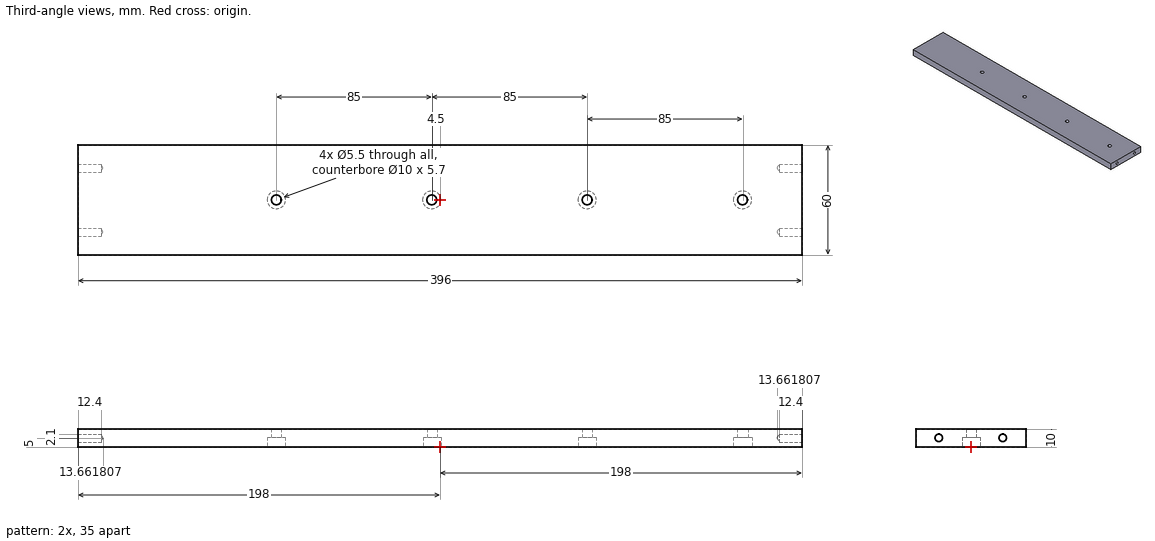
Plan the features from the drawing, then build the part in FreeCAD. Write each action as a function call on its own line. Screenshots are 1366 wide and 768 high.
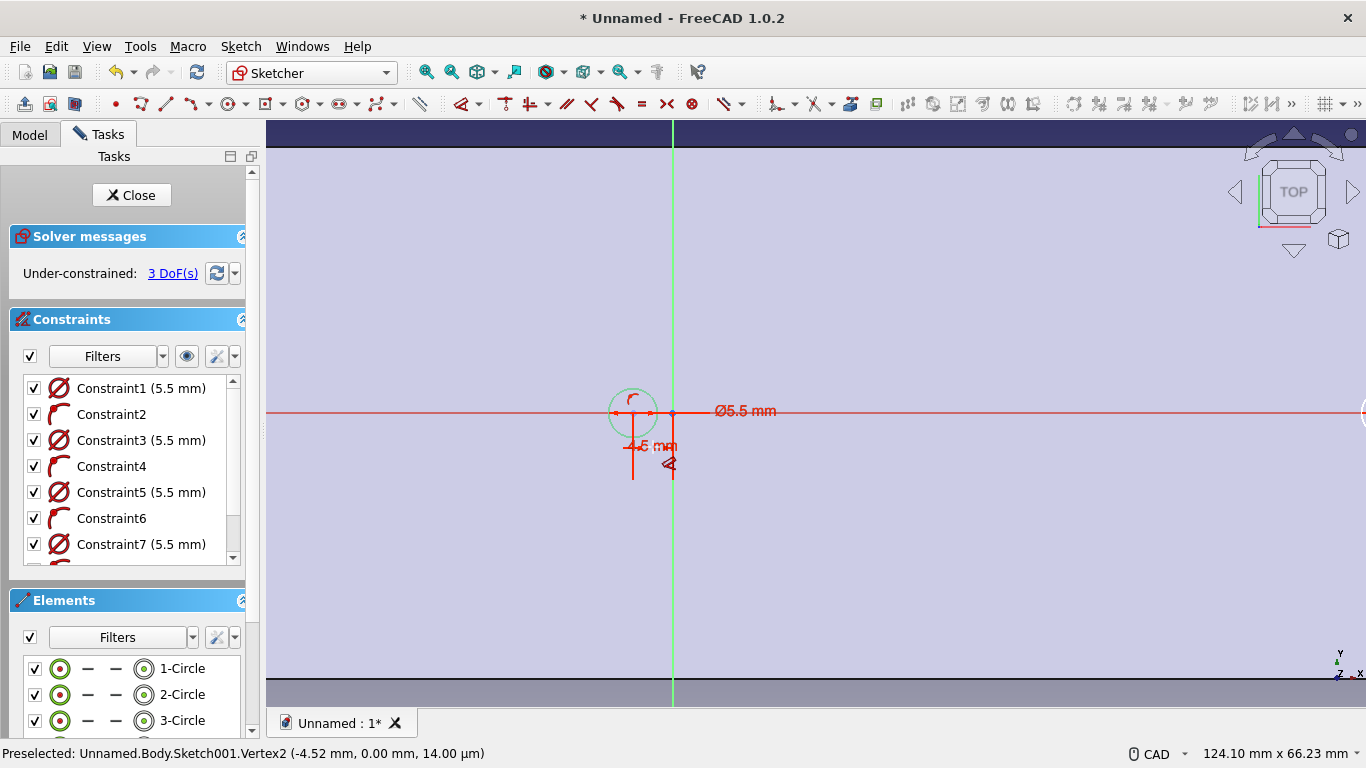
scroll(634, 414, down, 6)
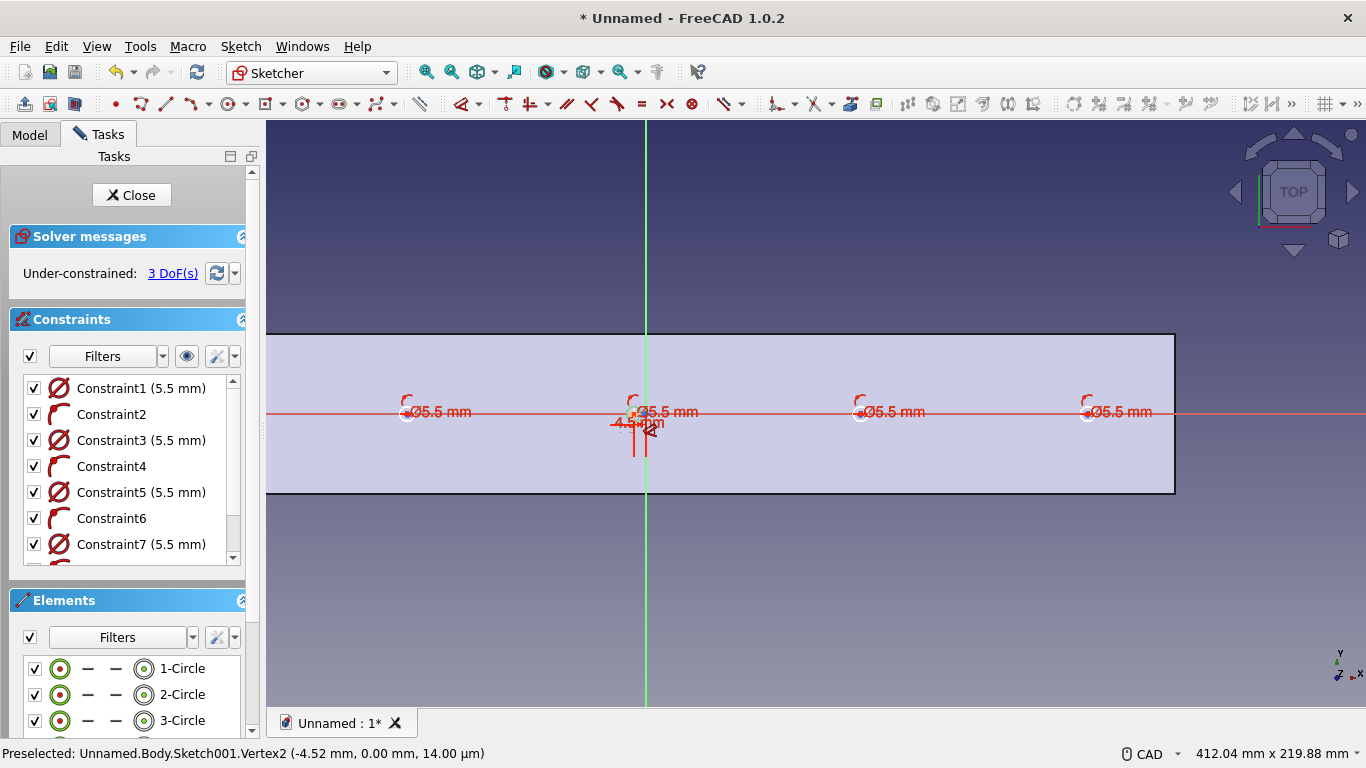
click(407, 414)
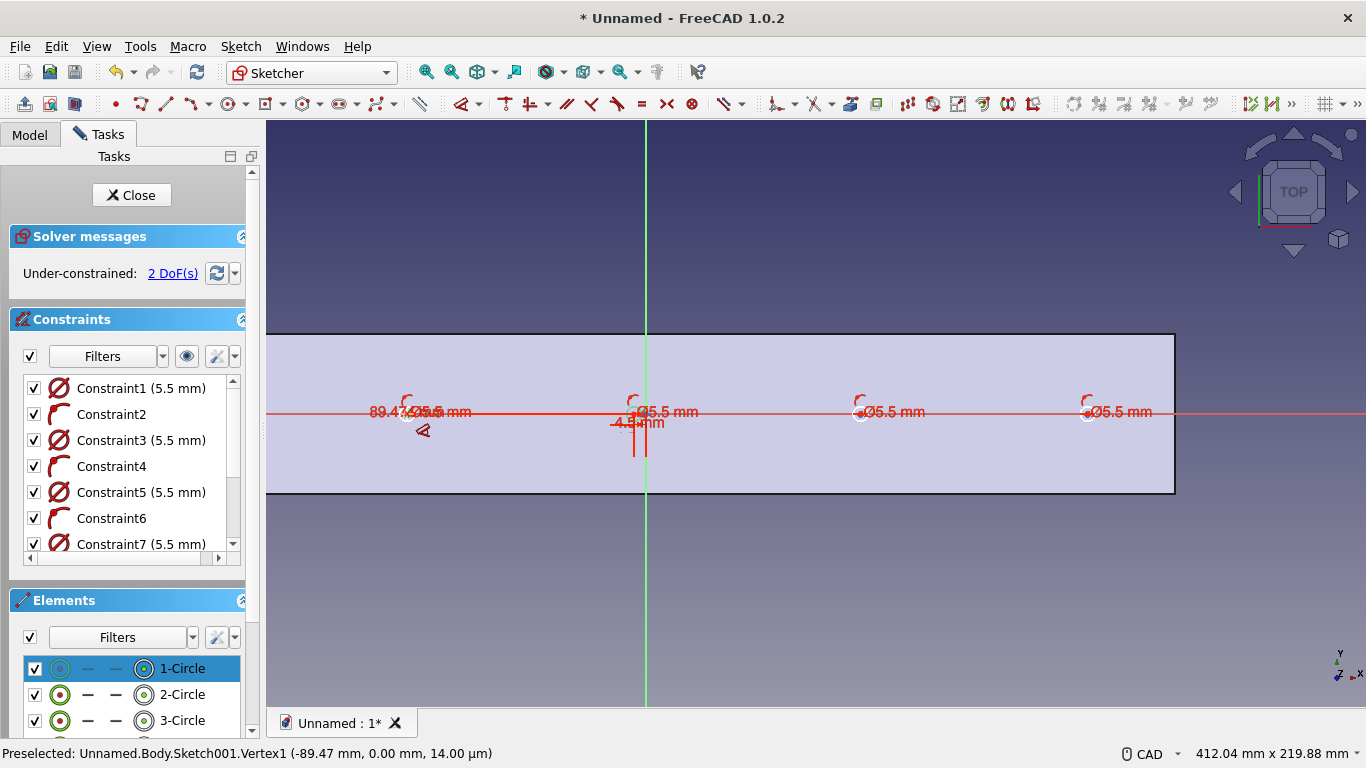
click(634, 414)
click(521, 448)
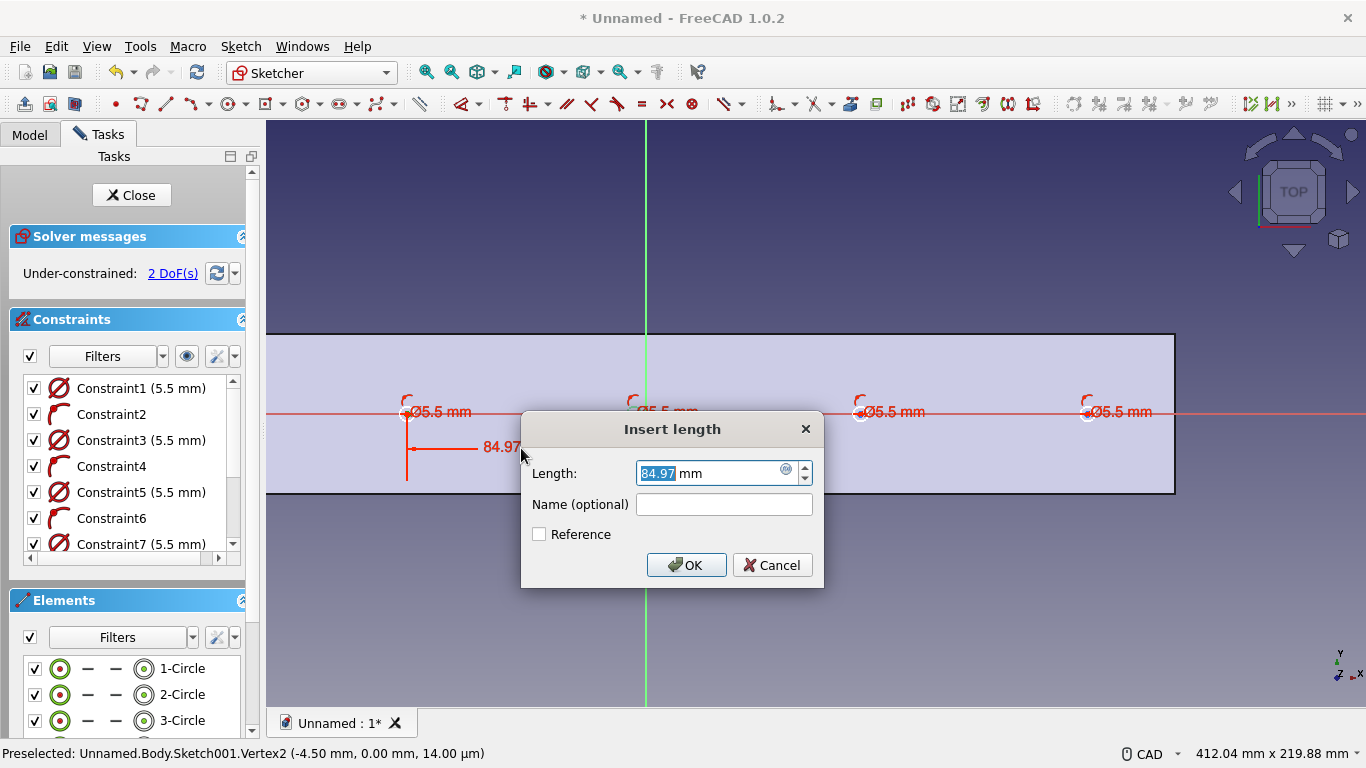
text(85)
key(Return)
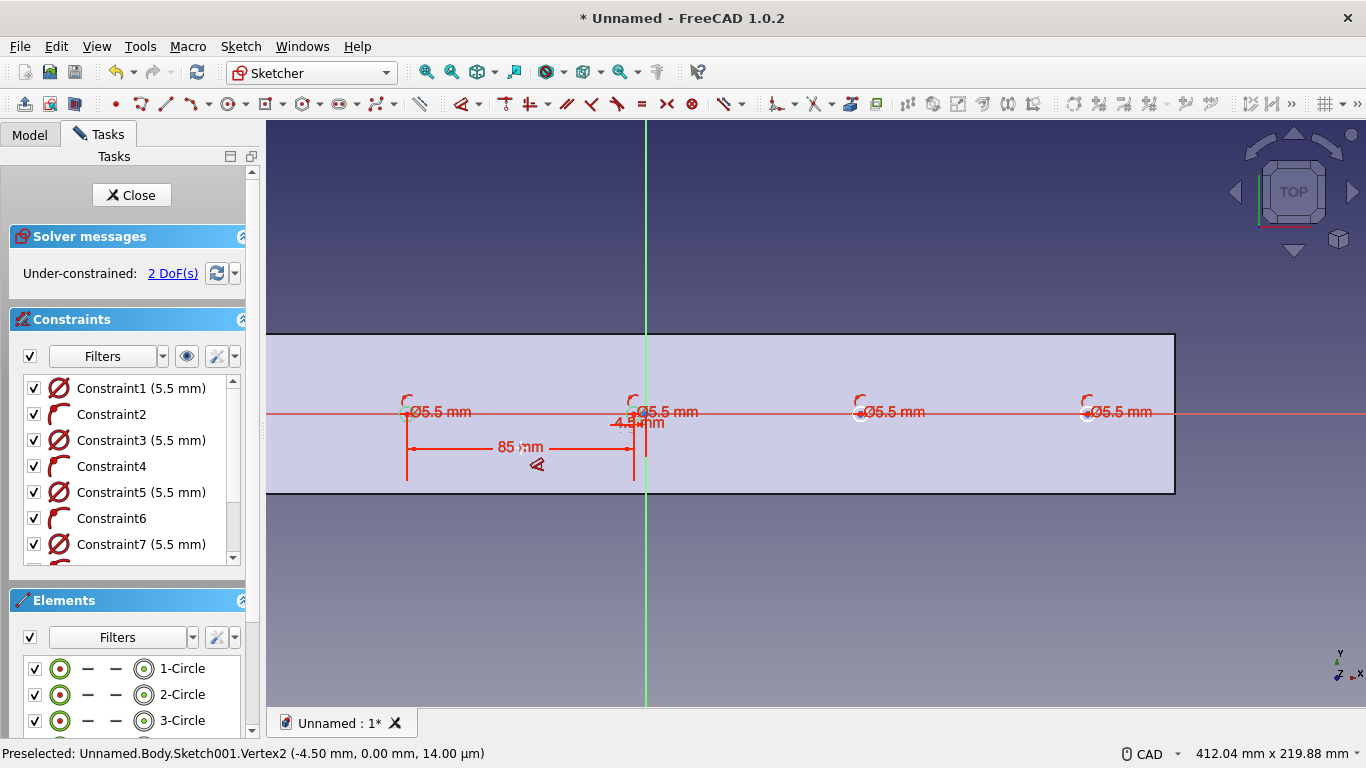
click(634, 414)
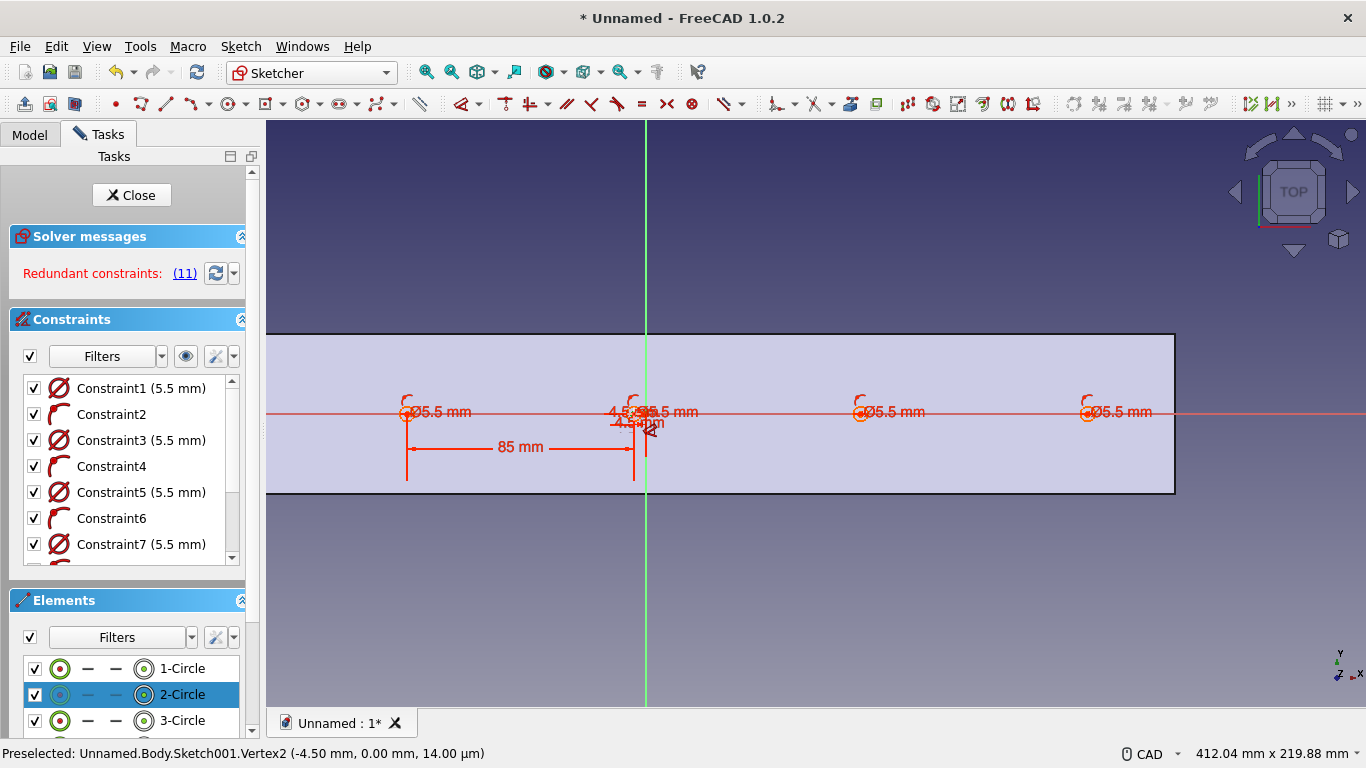
click(861, 414)
click(747, 448)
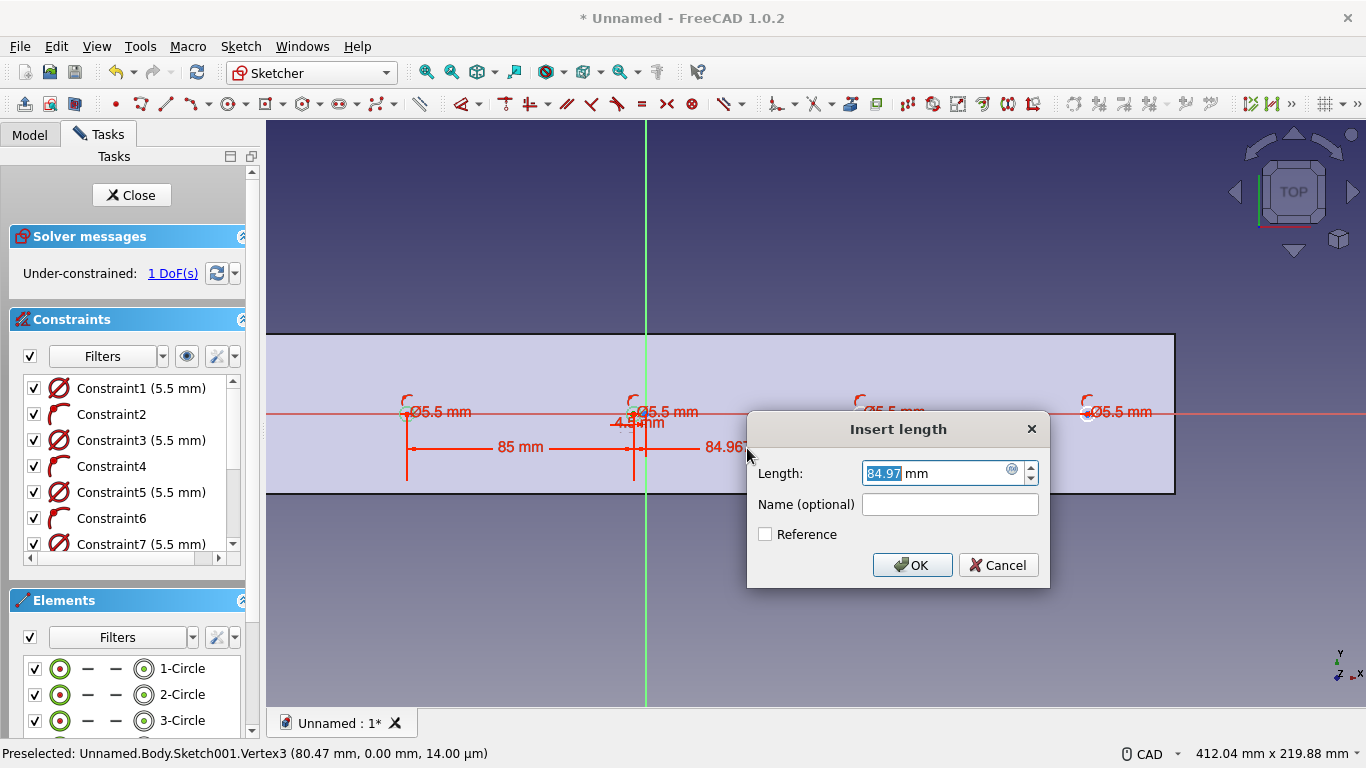
text(85)
key(Return)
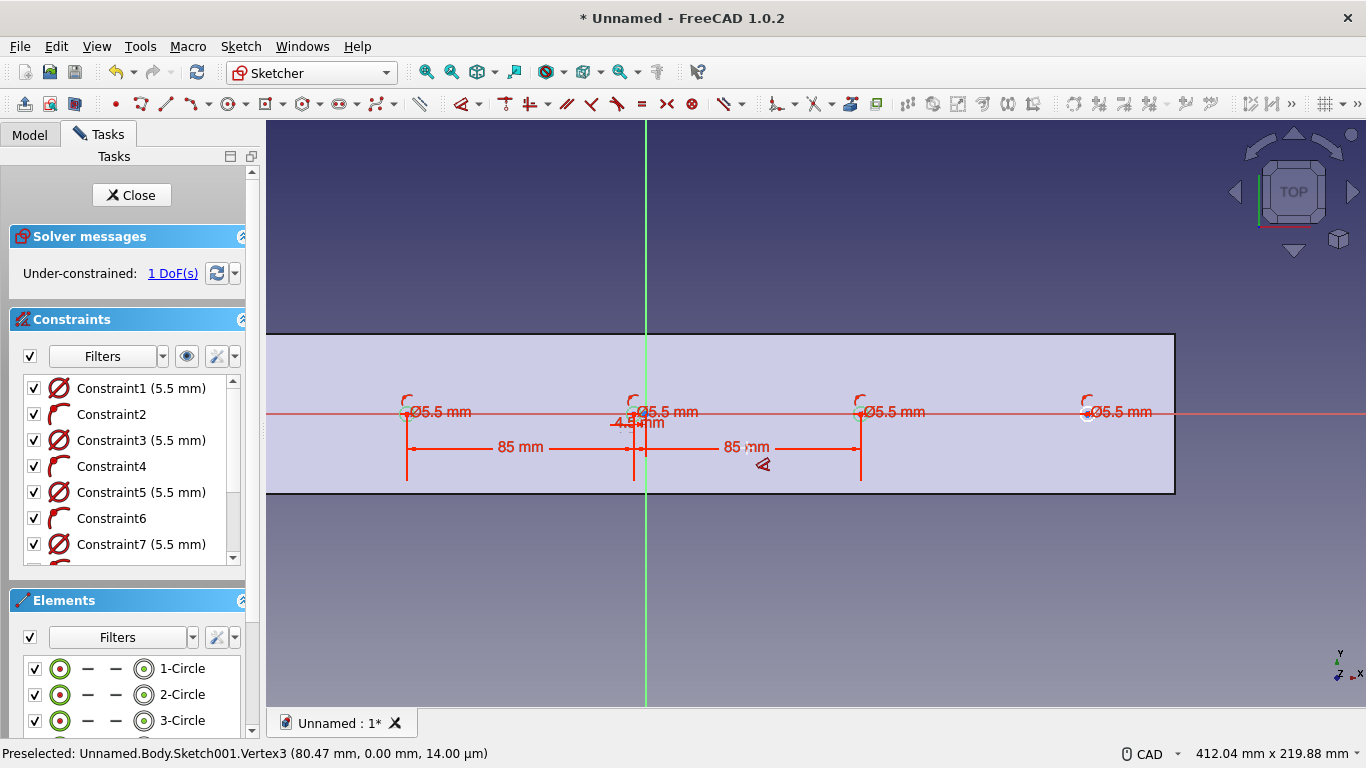
click(861, 414)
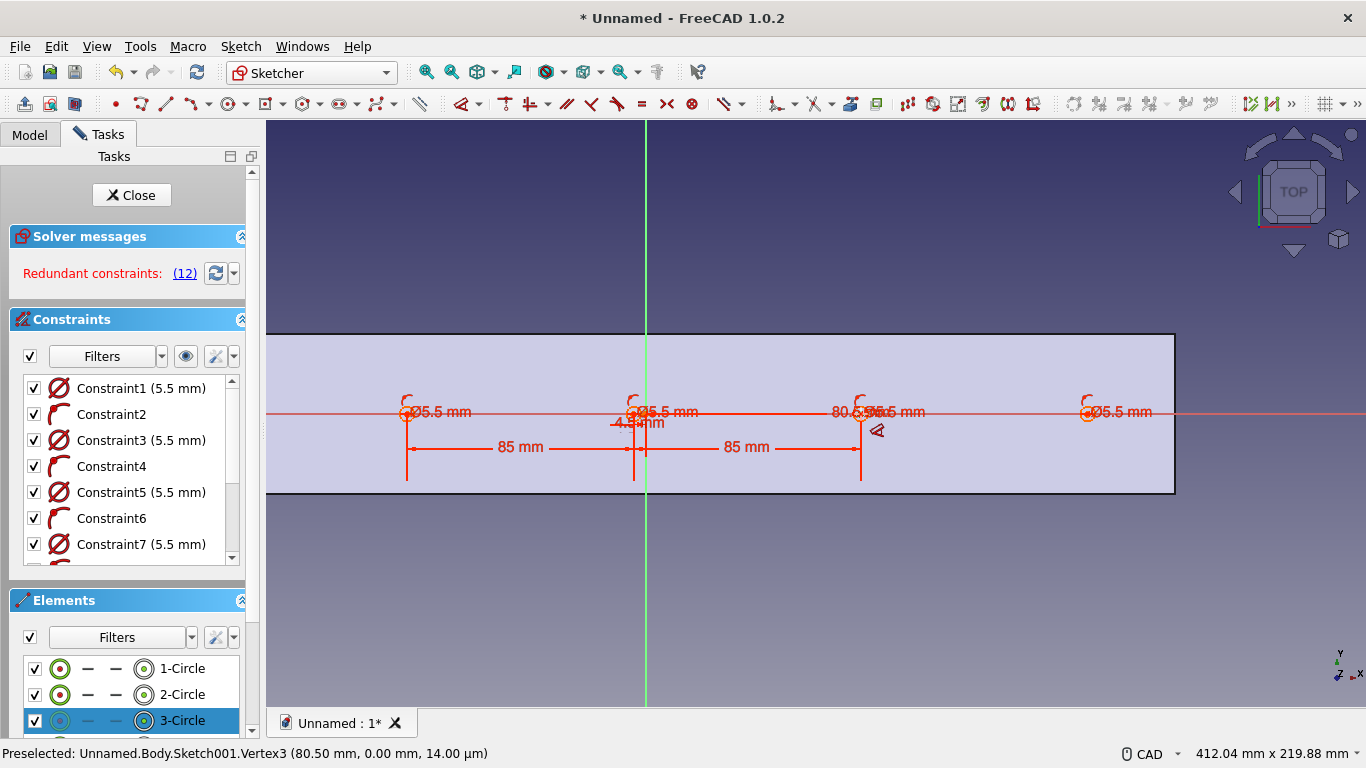
click(1088, 414)
click(974, 448)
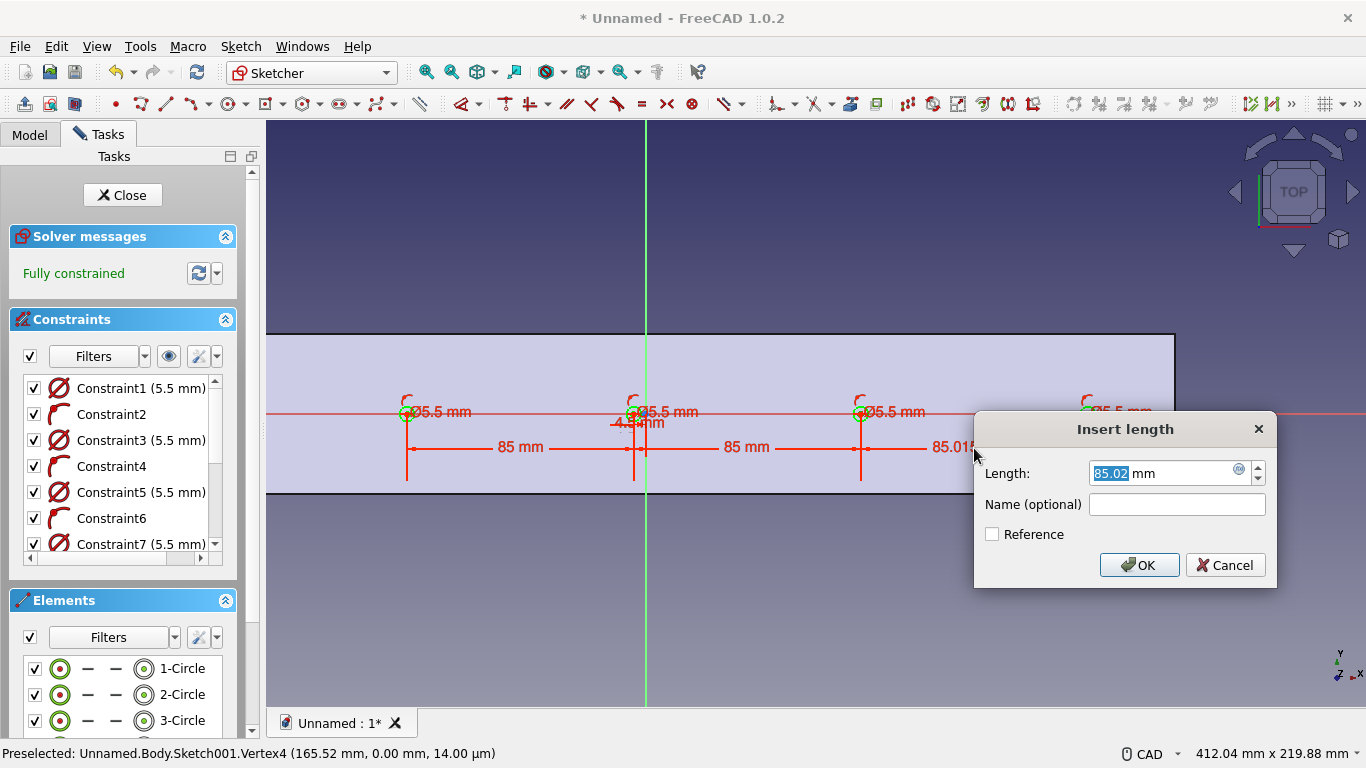
text(85)
key(Return)
key(Escape)